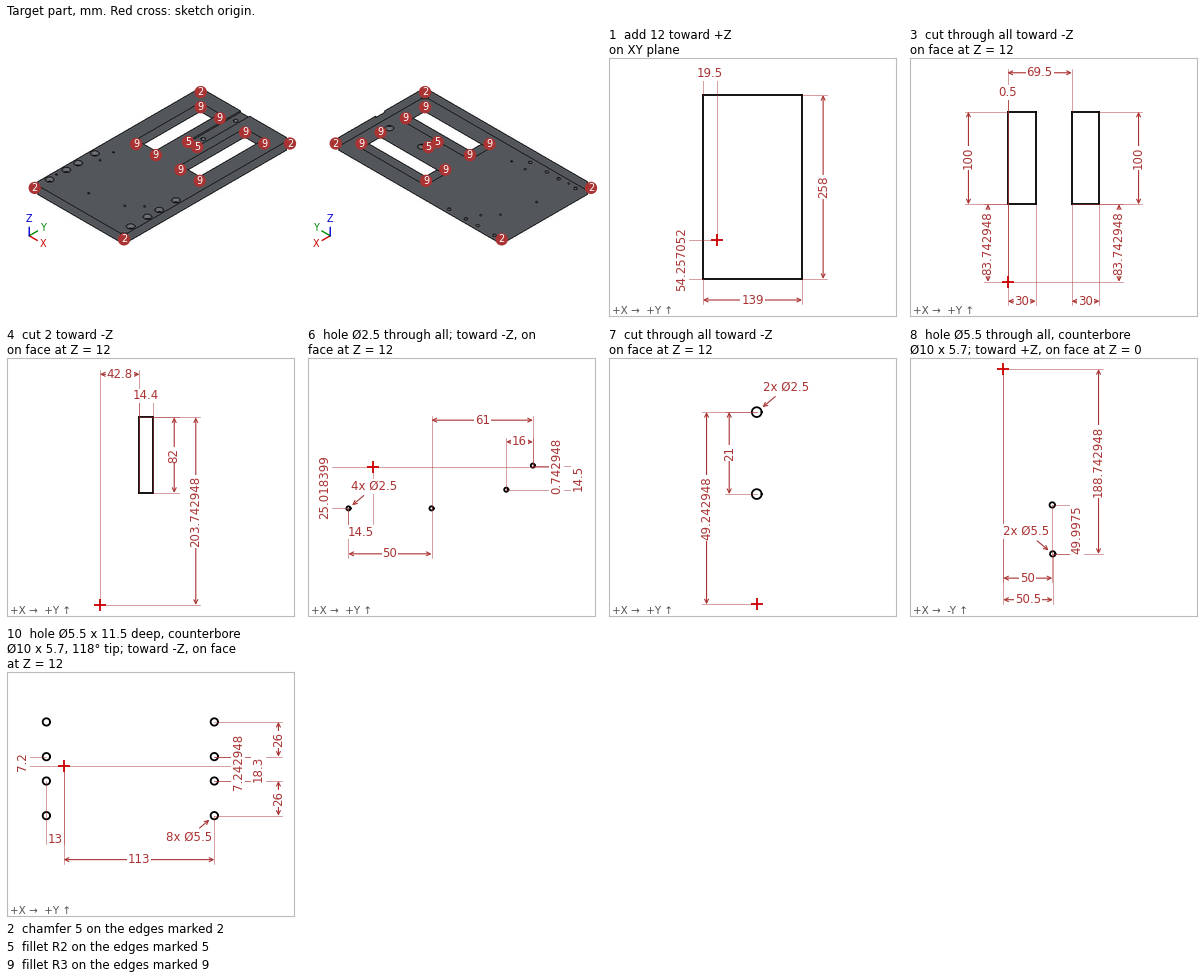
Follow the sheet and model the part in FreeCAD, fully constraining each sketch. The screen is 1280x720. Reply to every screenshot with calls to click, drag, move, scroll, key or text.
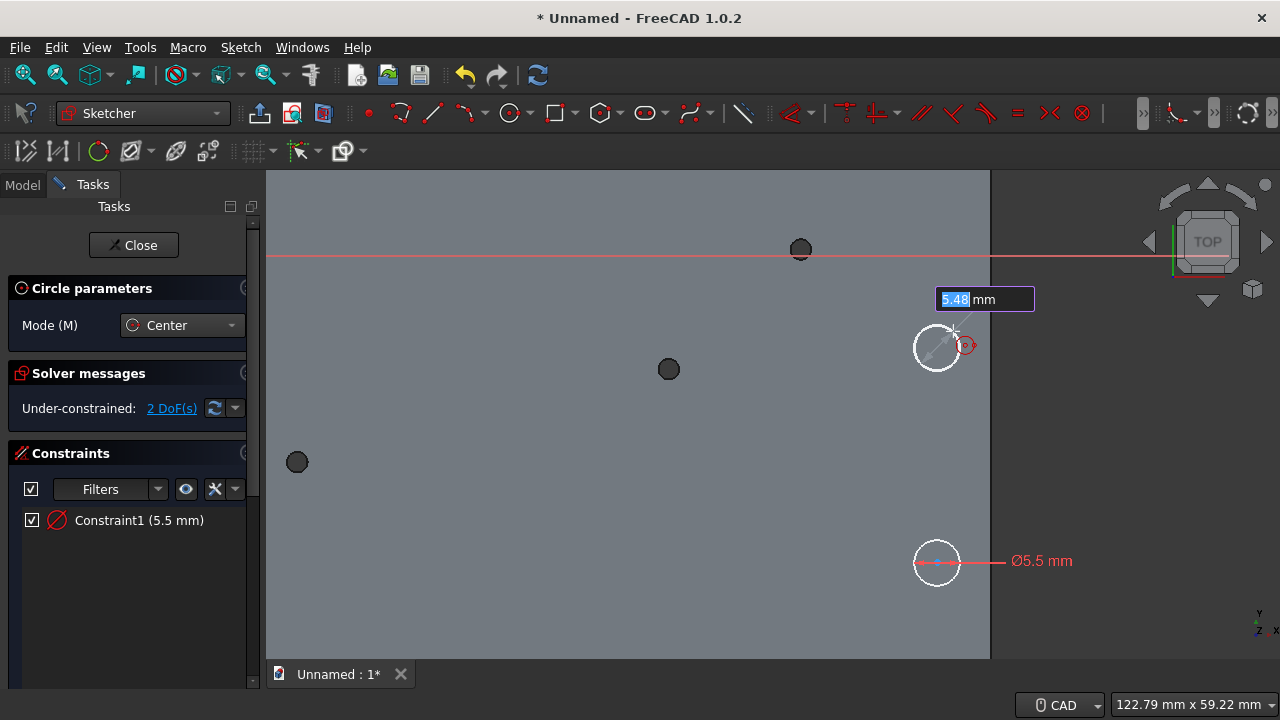
text(5.5)
key(Return)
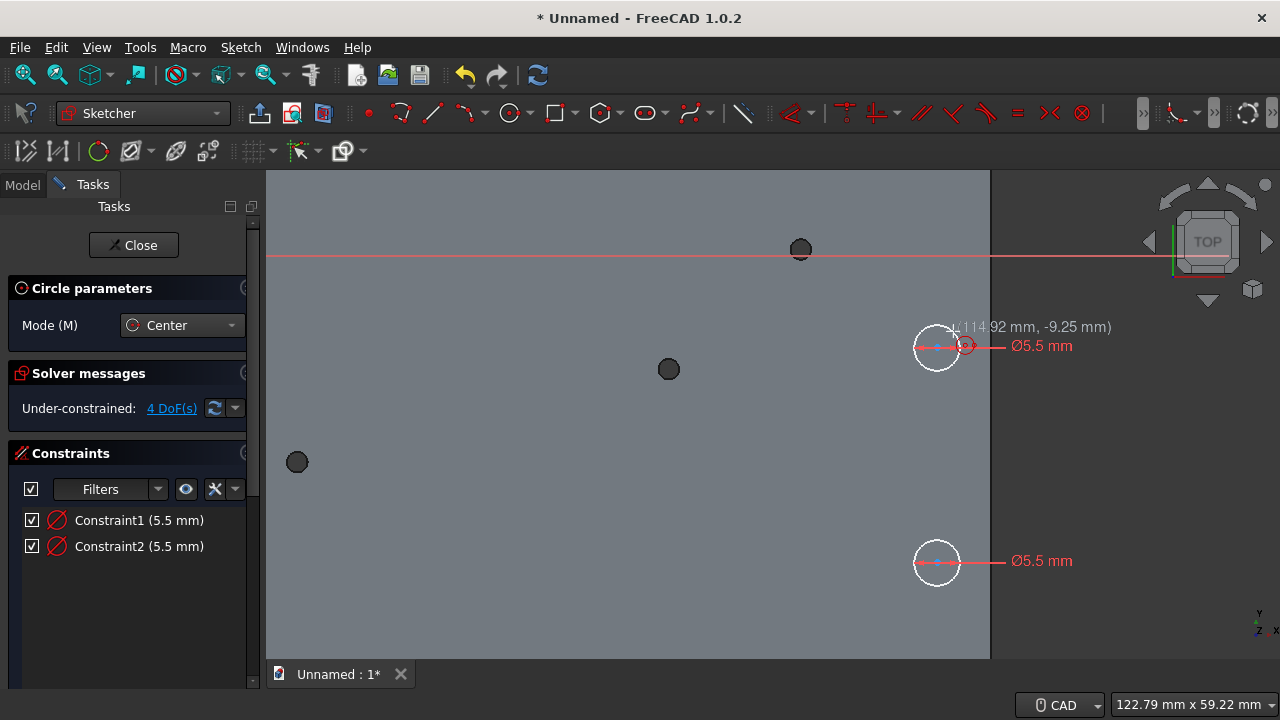
scroll(939, 531, down, 4)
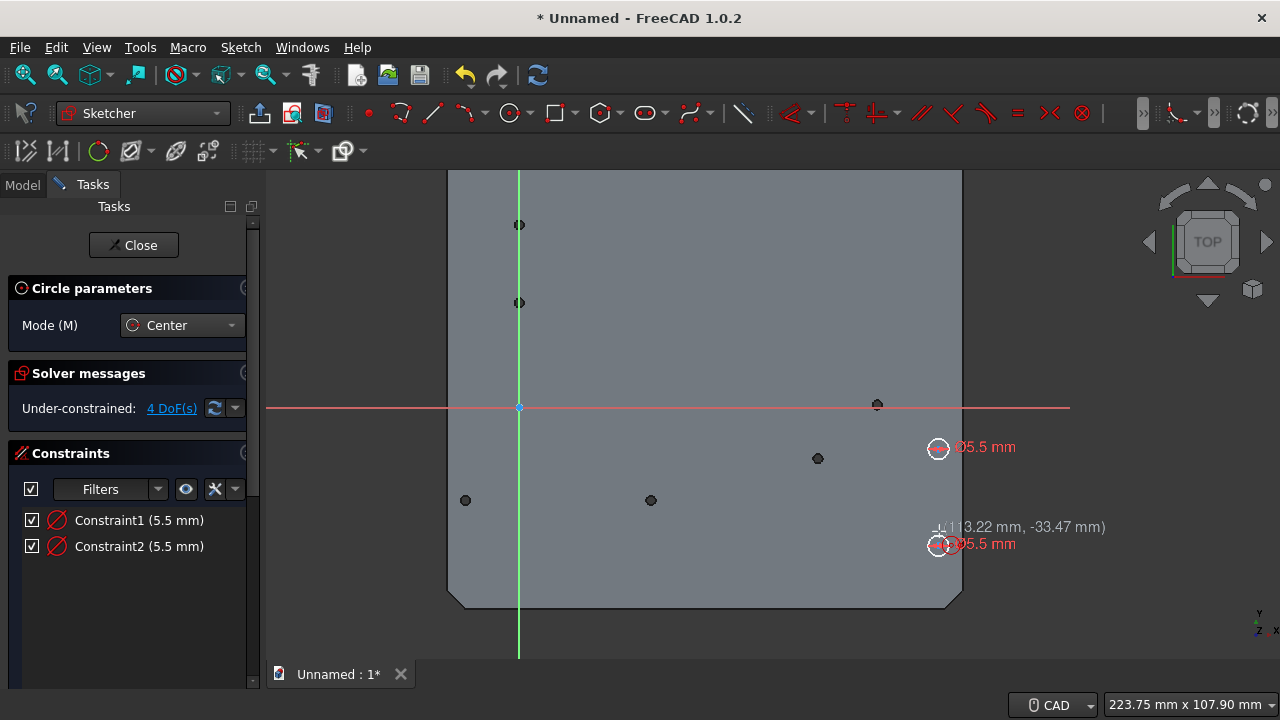
scroll(939, 381, up, 4)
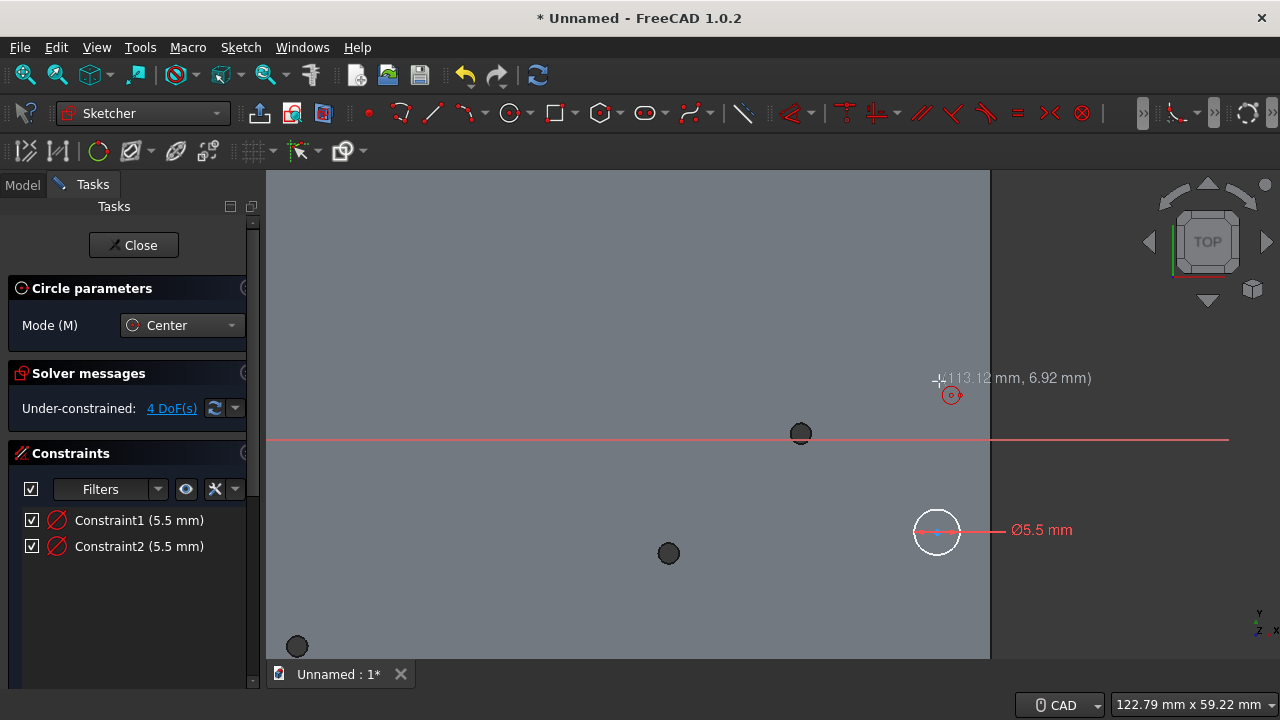
click(937, 380)
move(953, 364)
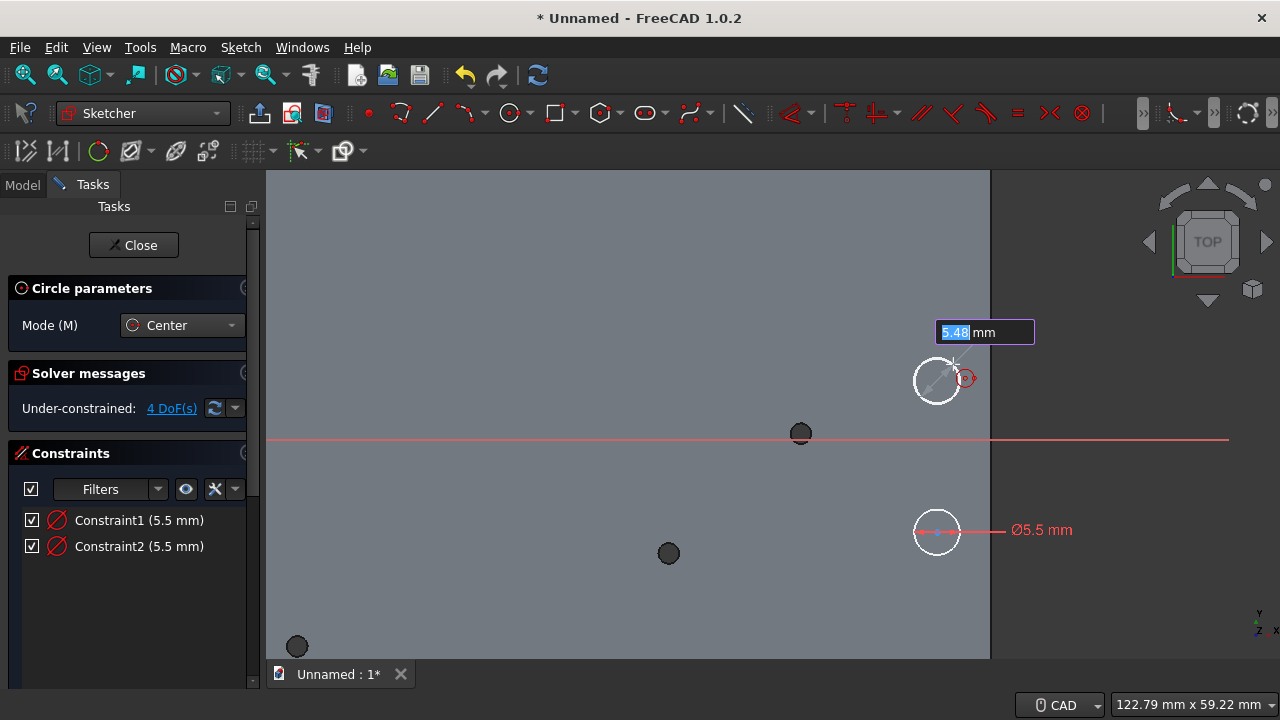
text(5.5)
key(Return)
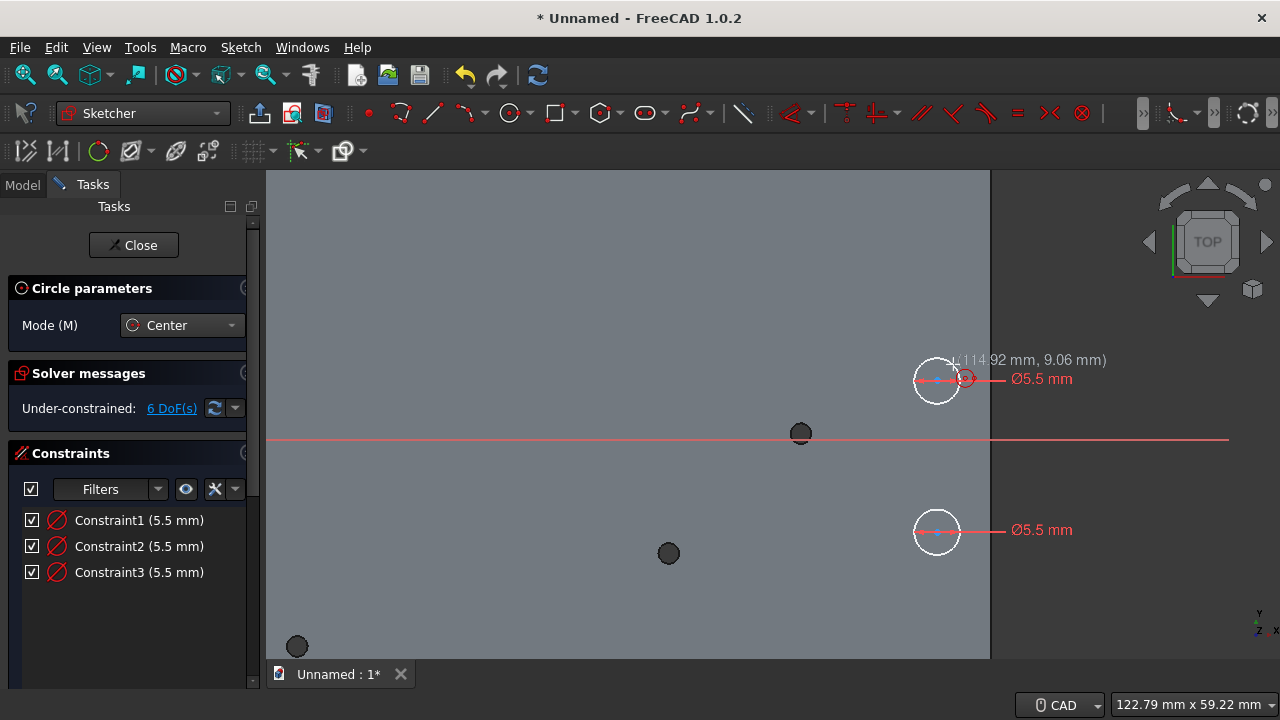
scroll(939, 381, down, 4)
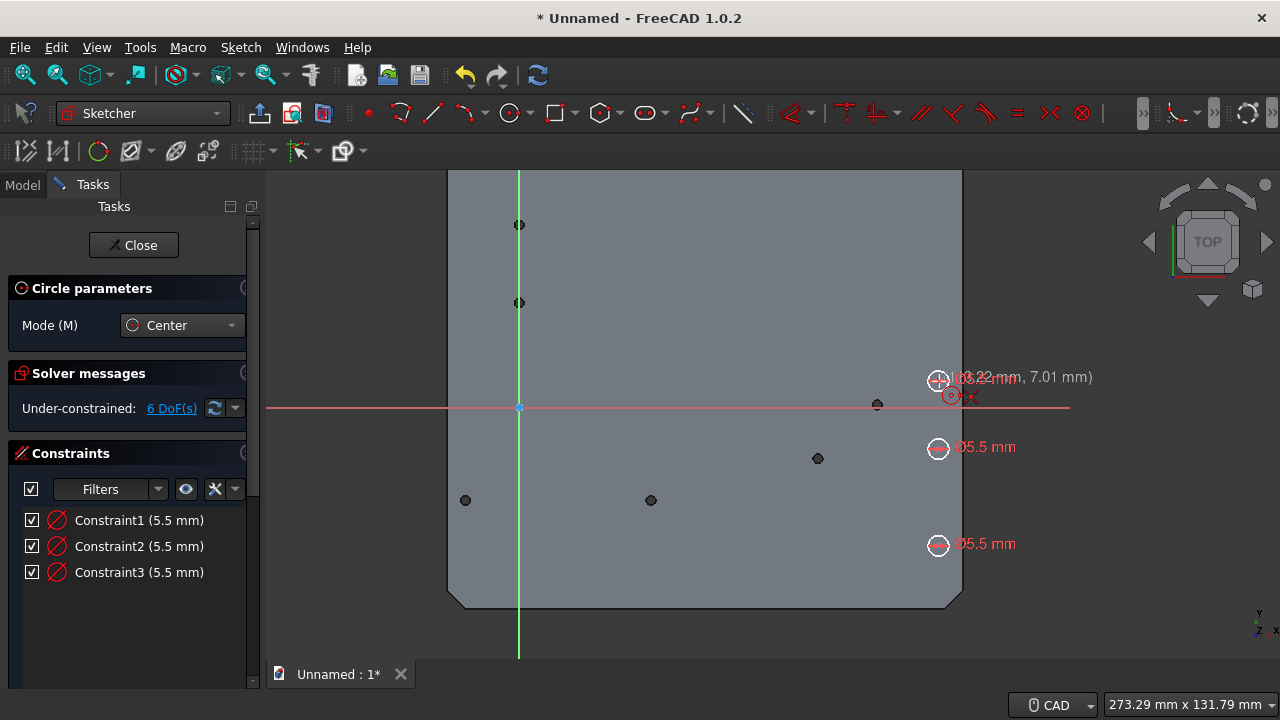
scroll(939, 284, up, 4)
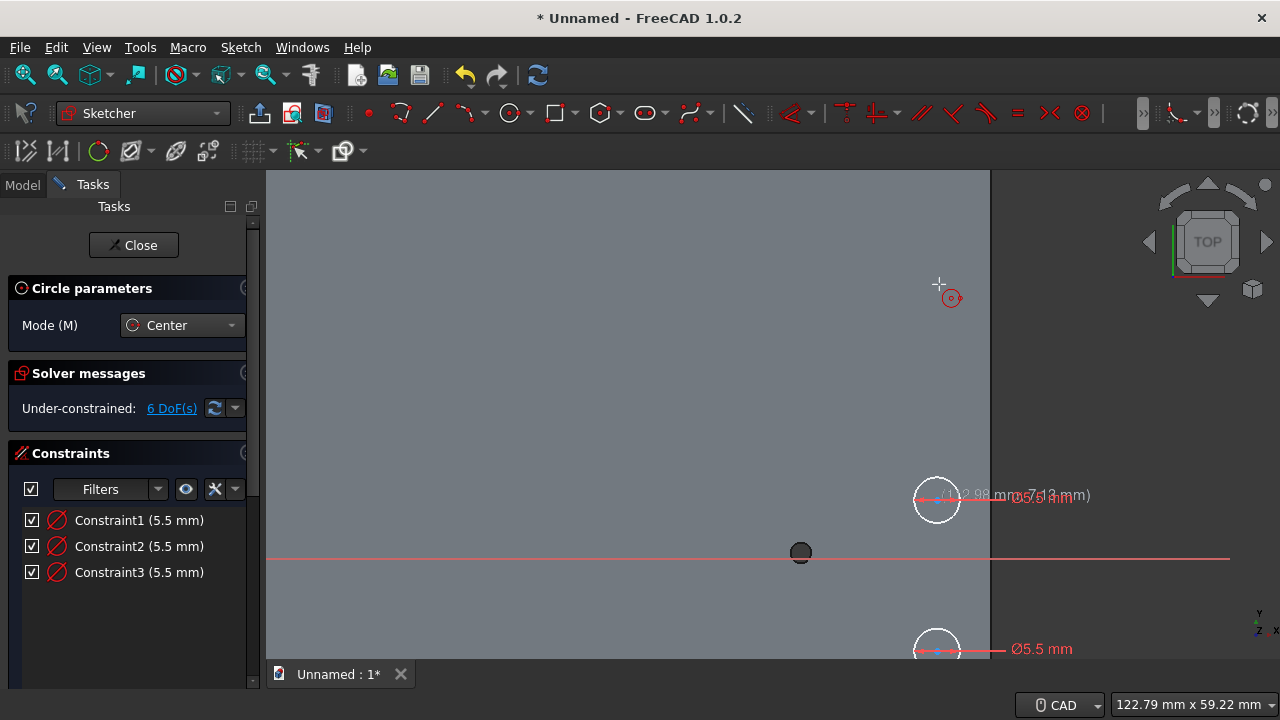
click(937, 284)
move(953, 268)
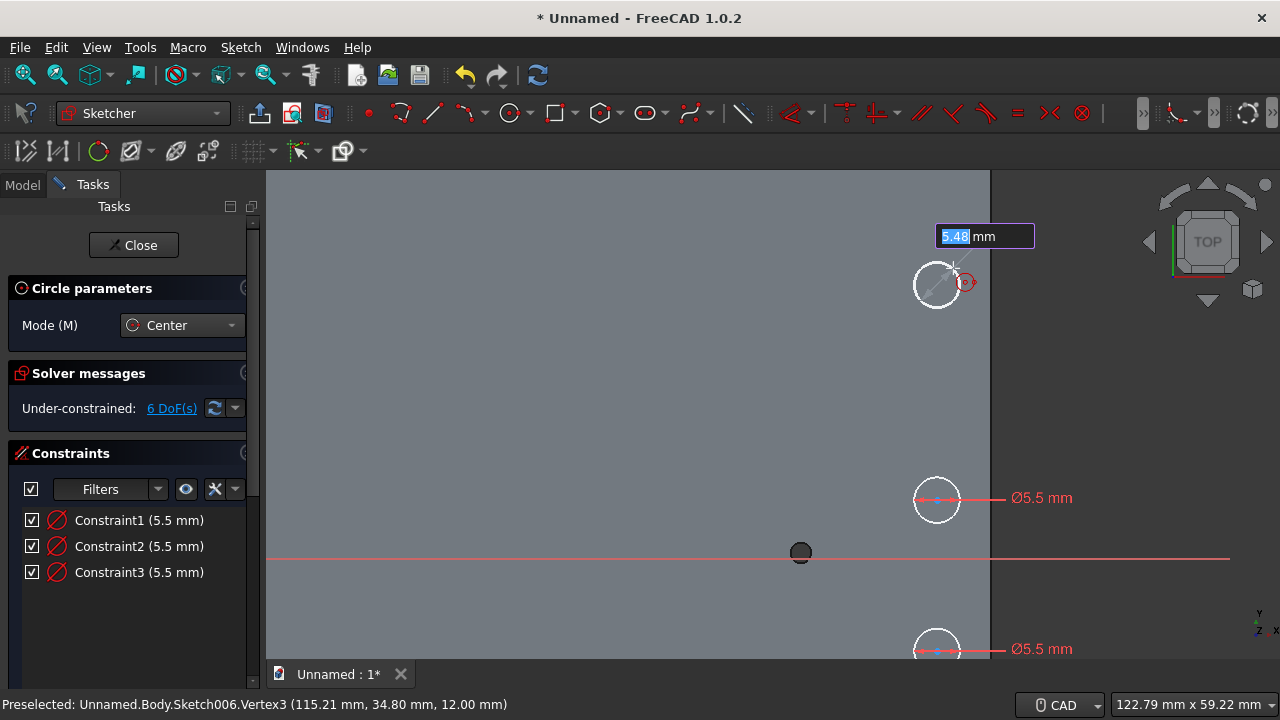
text(5.5)
key(Return)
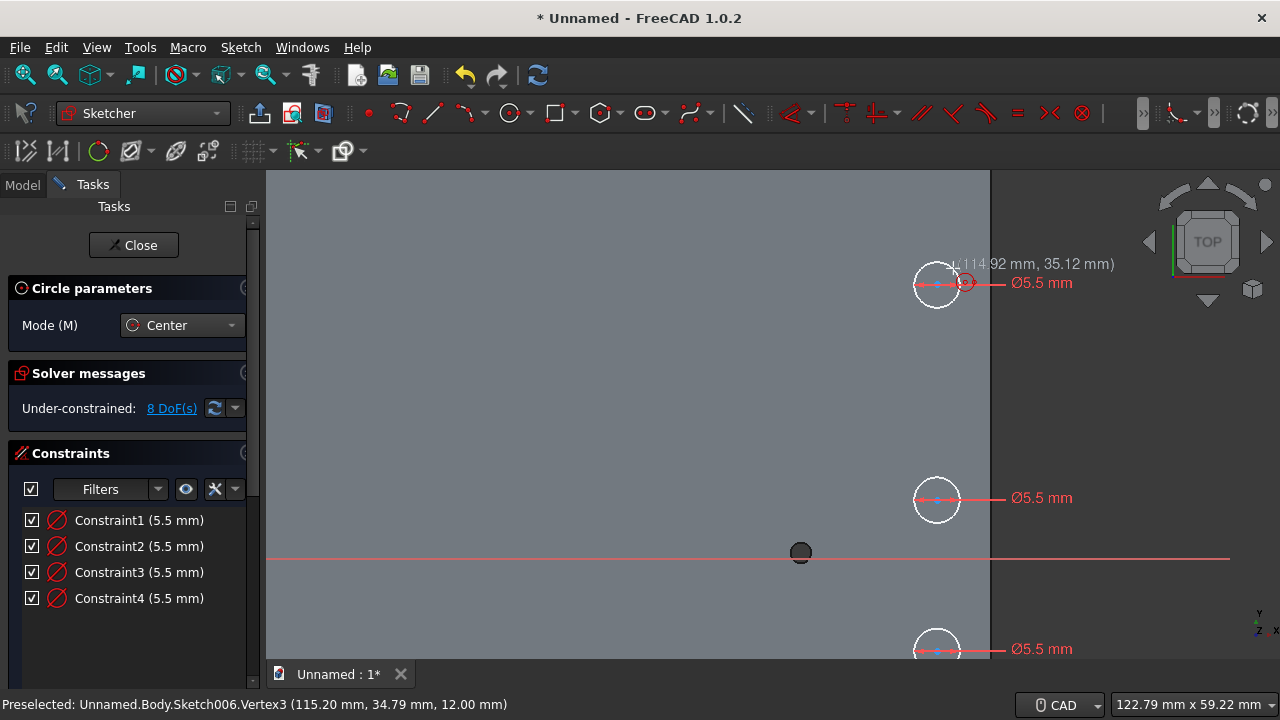
scroll(939, 284, down, 4)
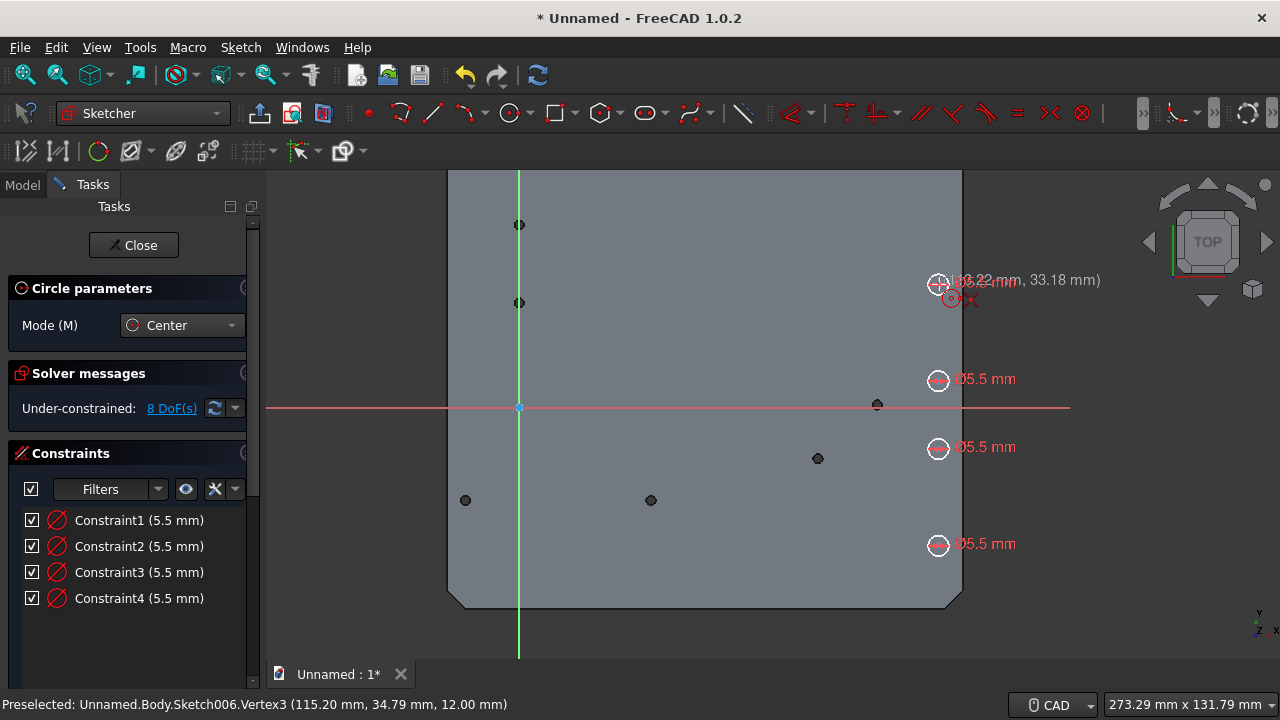
scroll(471, 449, up, 4)